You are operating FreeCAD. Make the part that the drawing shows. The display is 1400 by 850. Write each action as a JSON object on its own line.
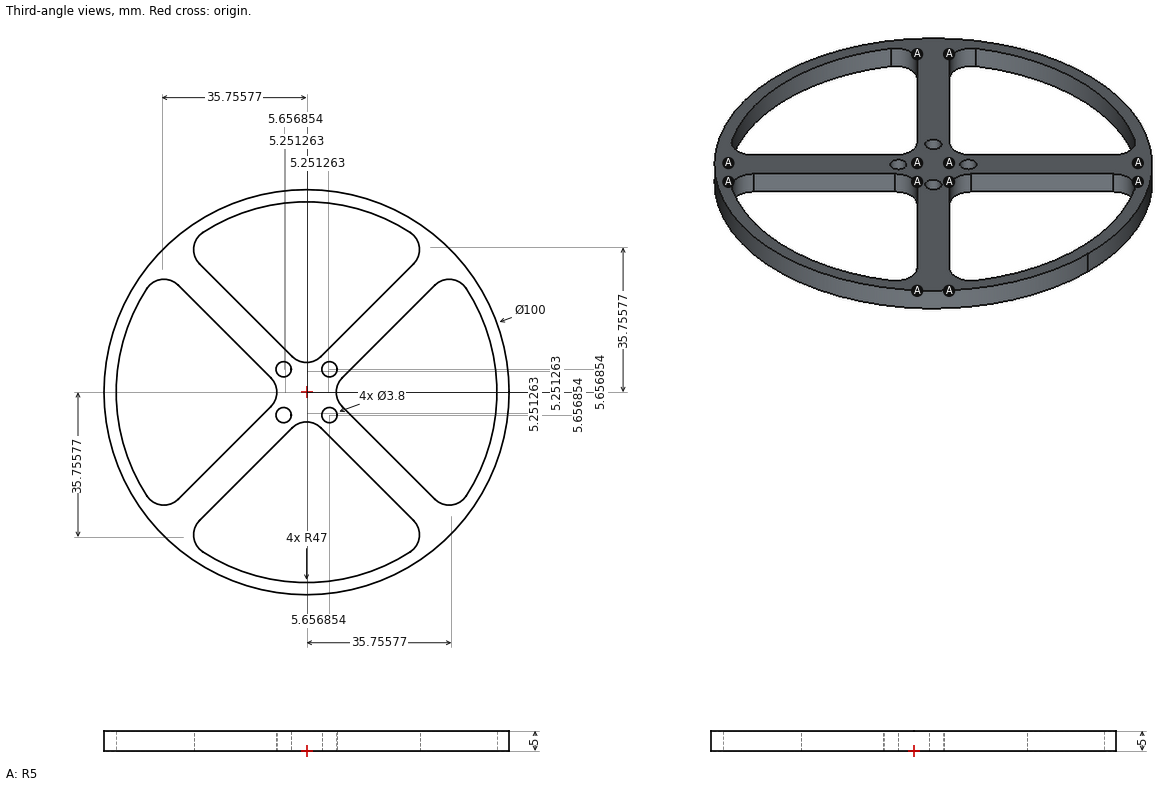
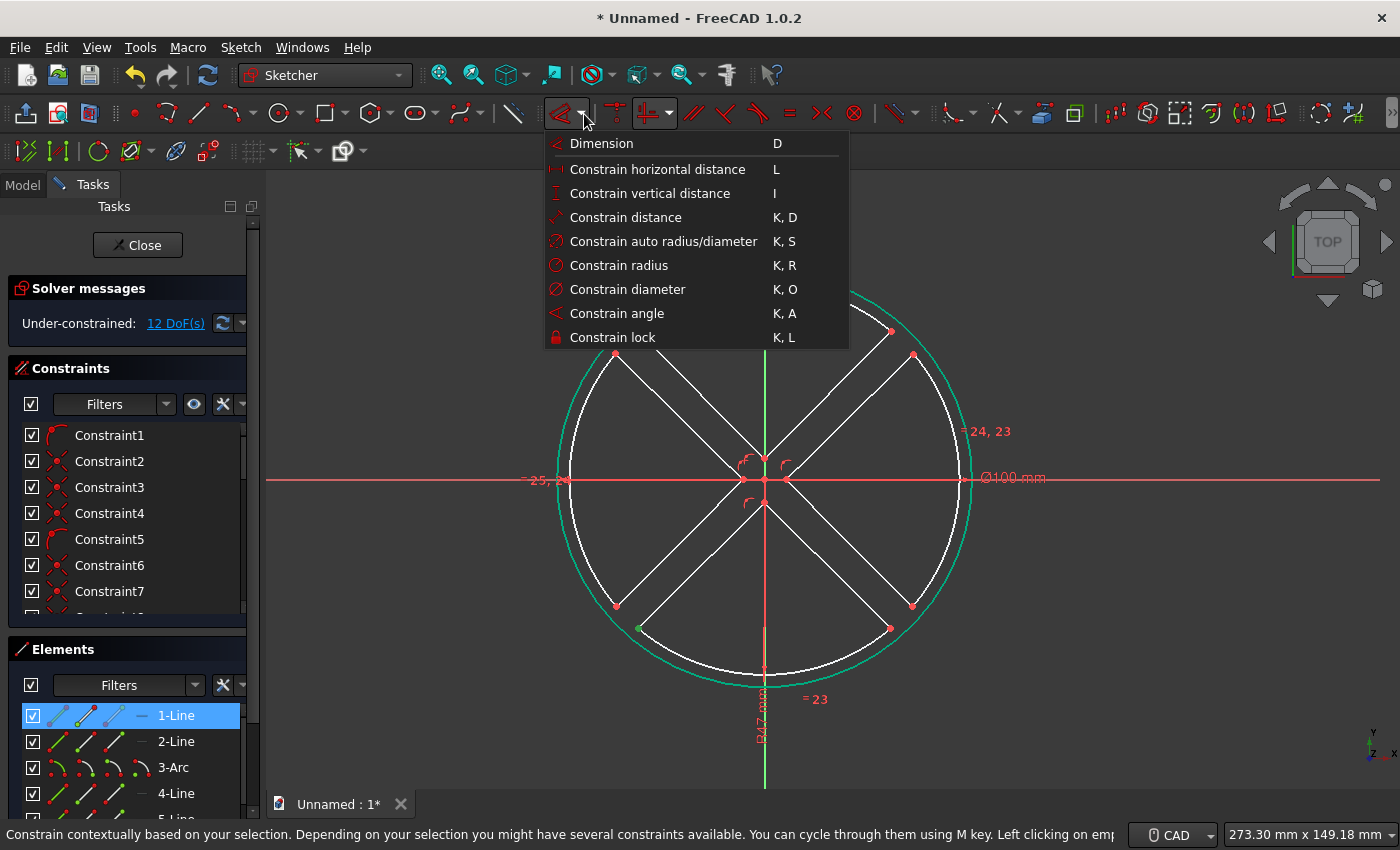
{"action": "left_click", "coordinate": [697, 193]}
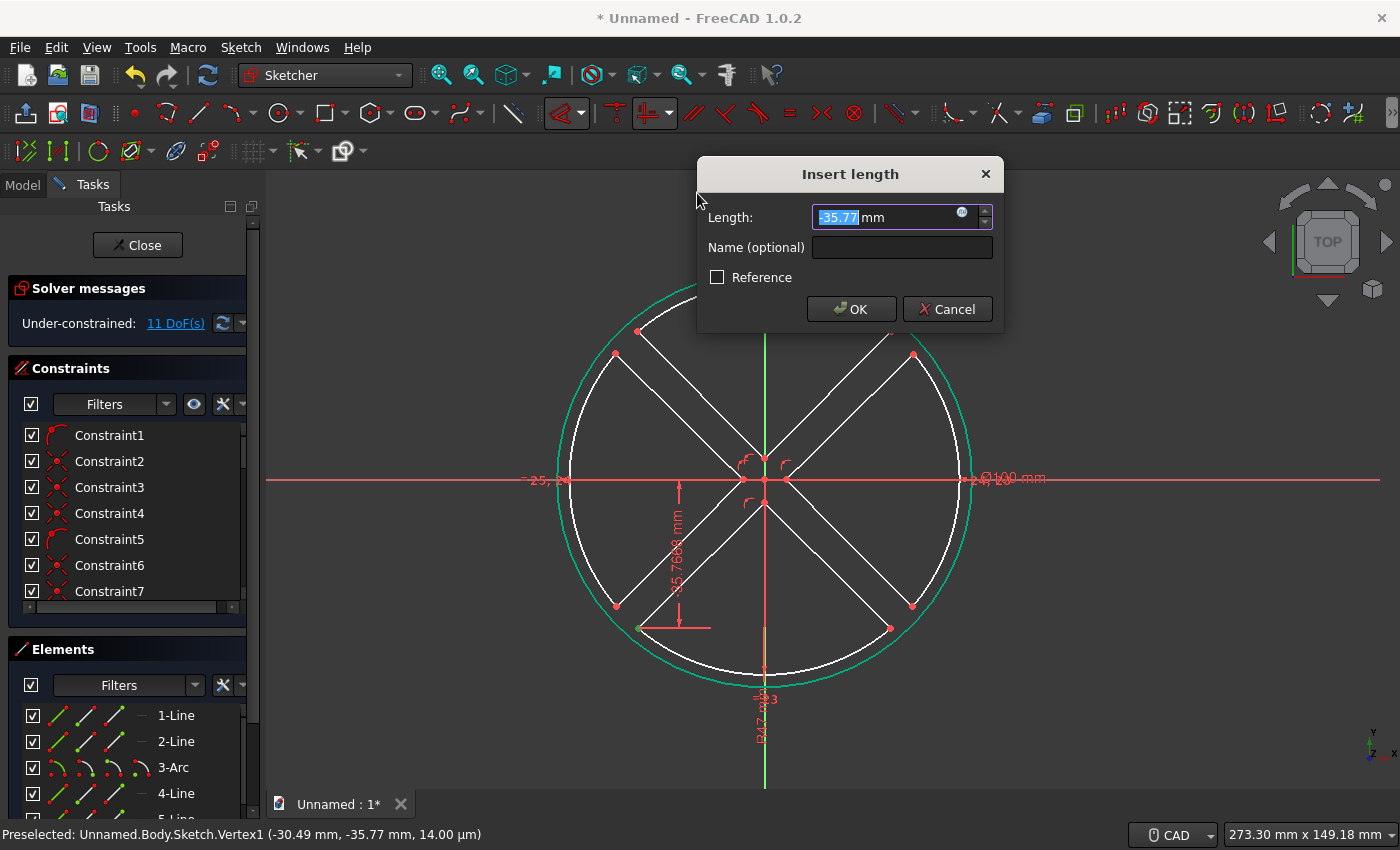
{"action": "type", "text": "-35.75577"}
{"action": "key", "text": "Return"}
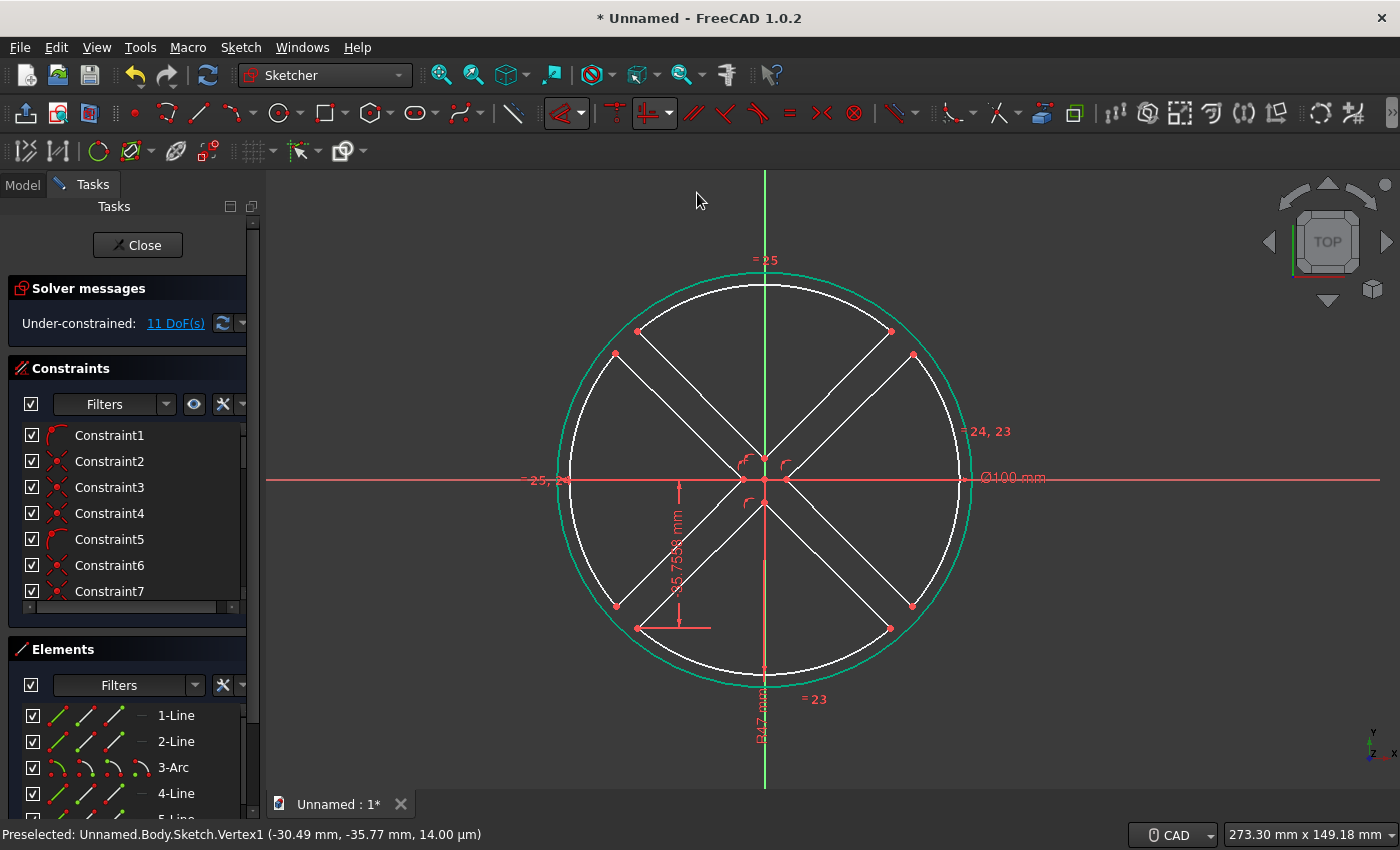
{"action": "scroll", "coordinate": [765, 503], "scroll_direction": "up", "scroll_amount": 3}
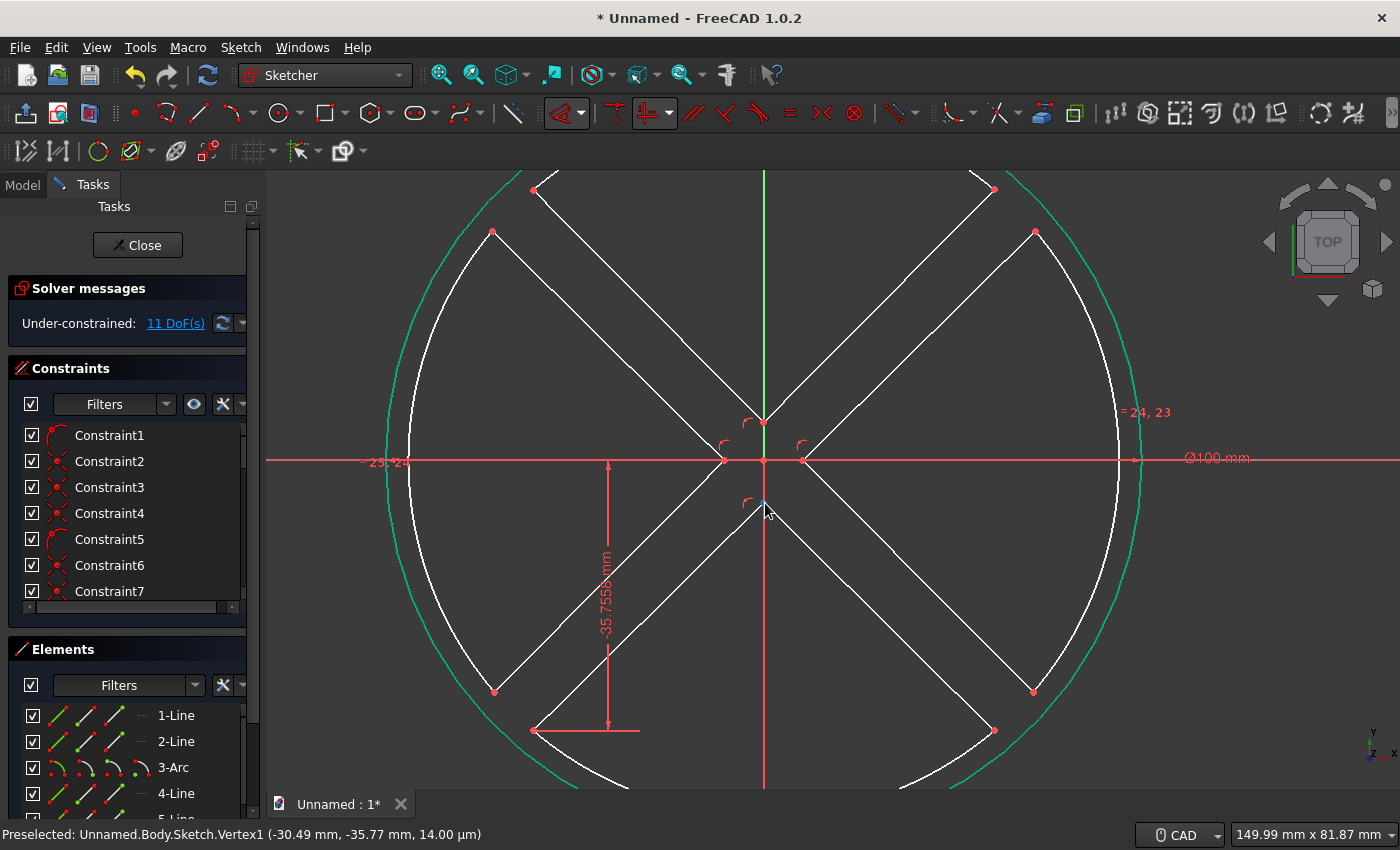
{"action": "left_click", "coordinate": [764, 503]}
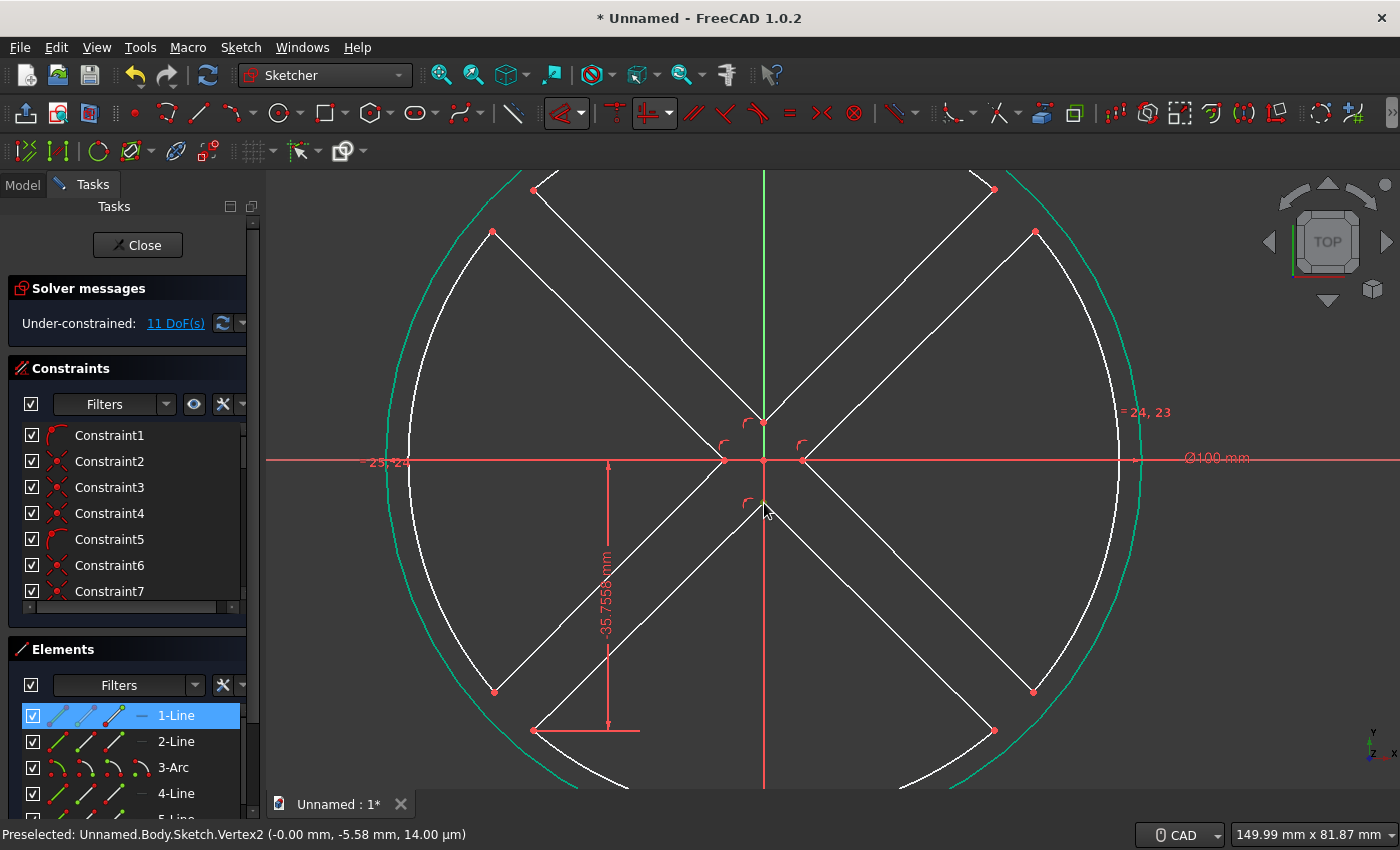
{"action": "key", "text": "i"}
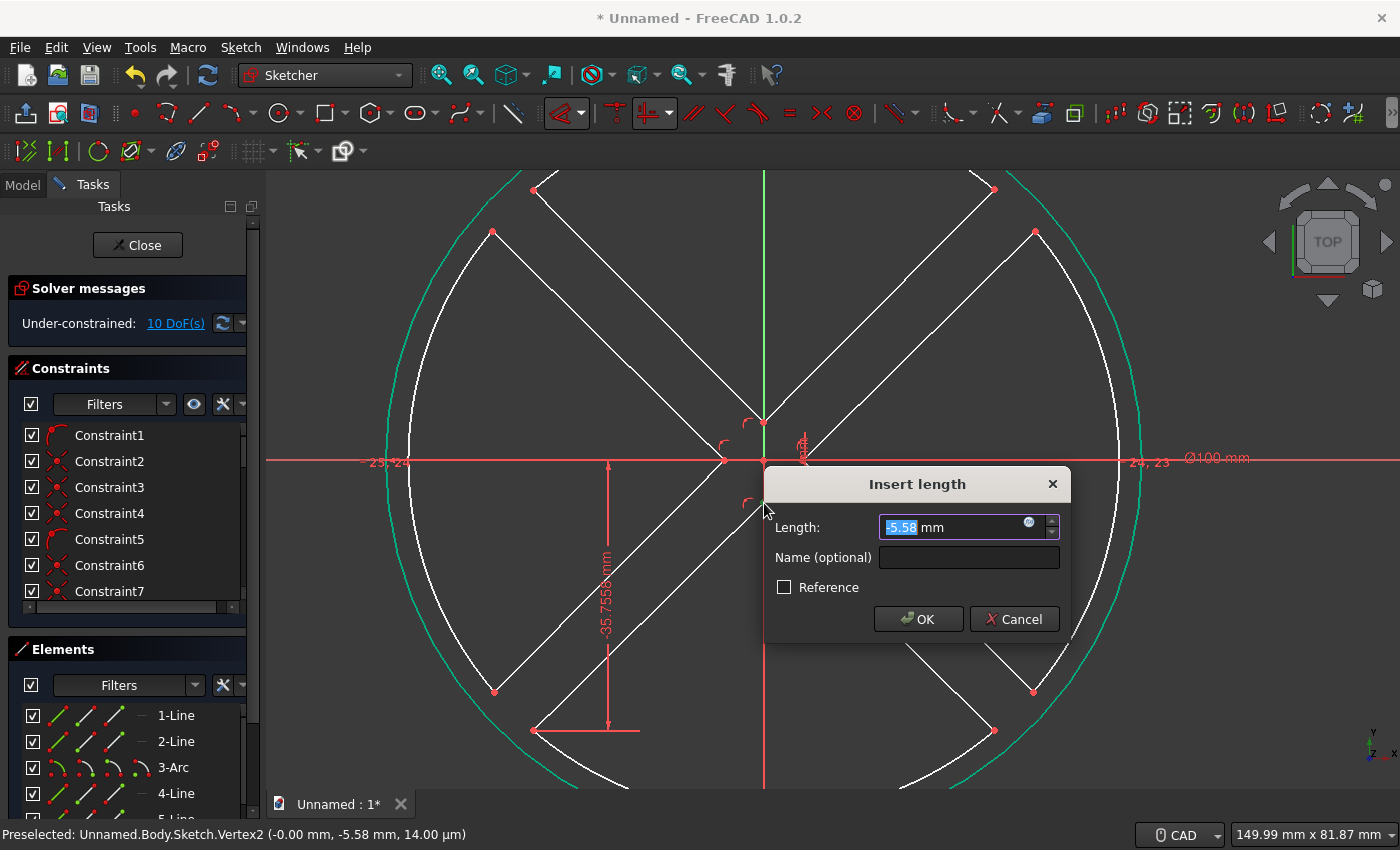
{"action": "type", "text": "-5.251263"}
{"action": "key", "text": "Return"}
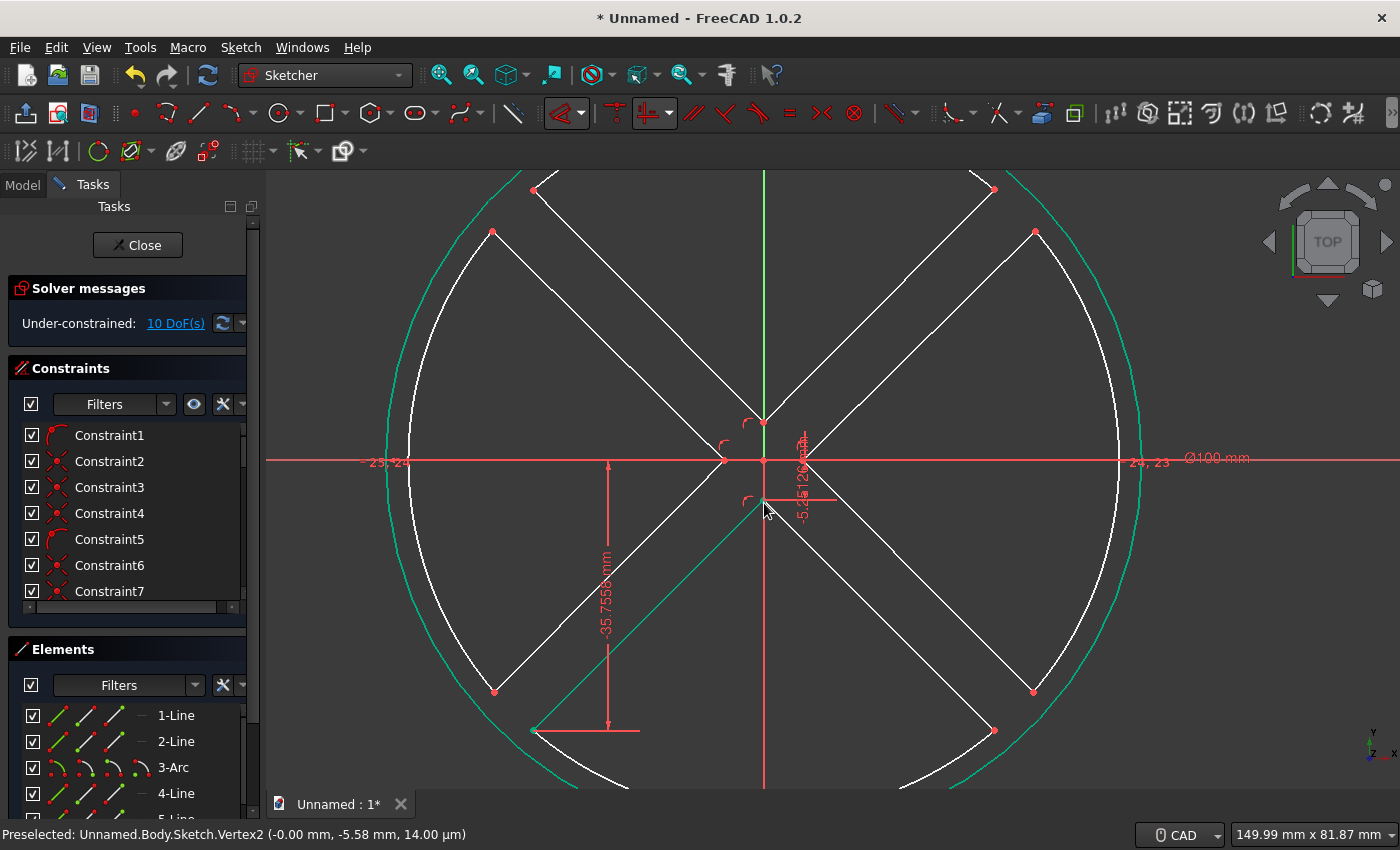
{"action": "left_click", "coordinate": [994, 731]}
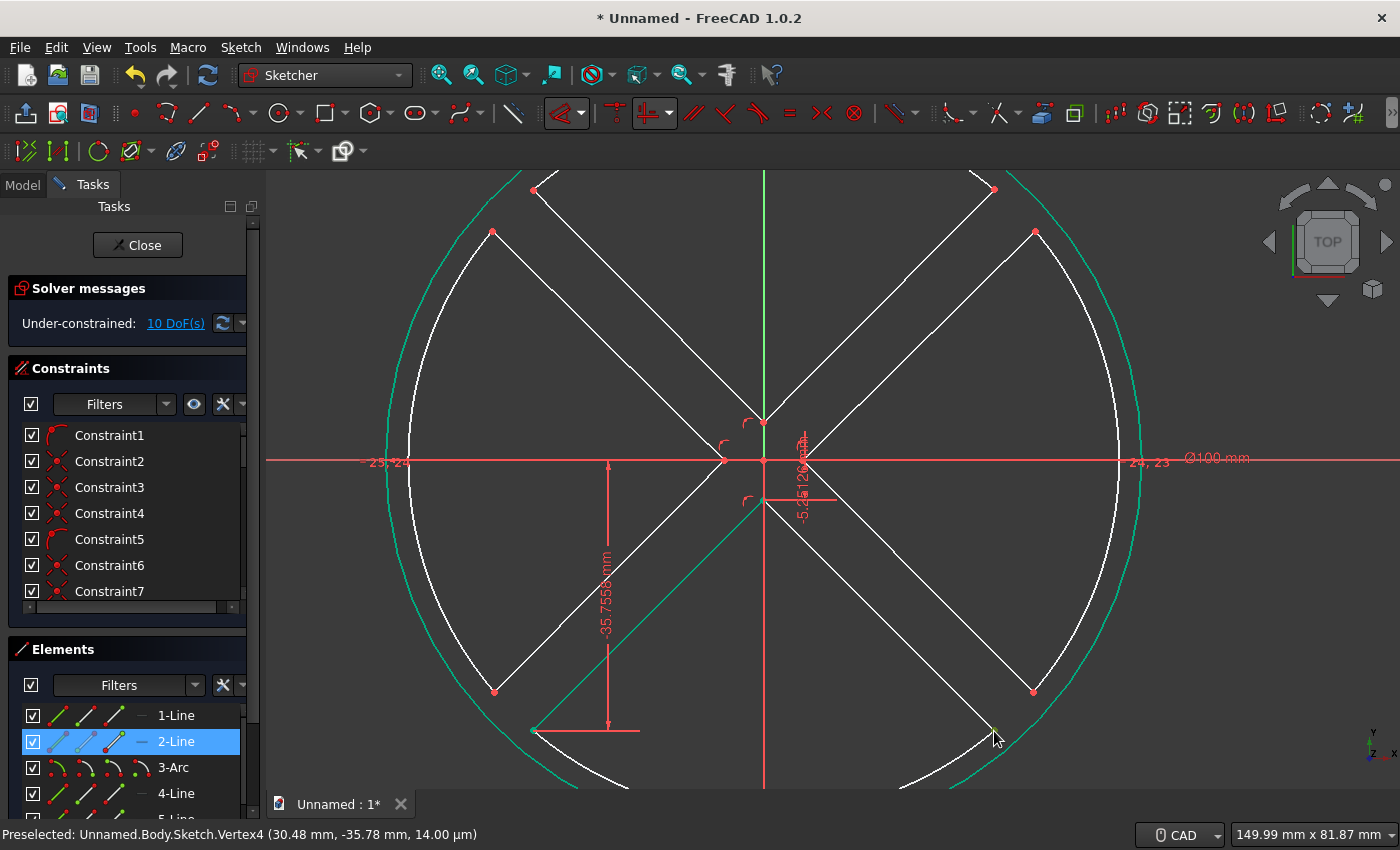
{"action": "key", "text": "i"}